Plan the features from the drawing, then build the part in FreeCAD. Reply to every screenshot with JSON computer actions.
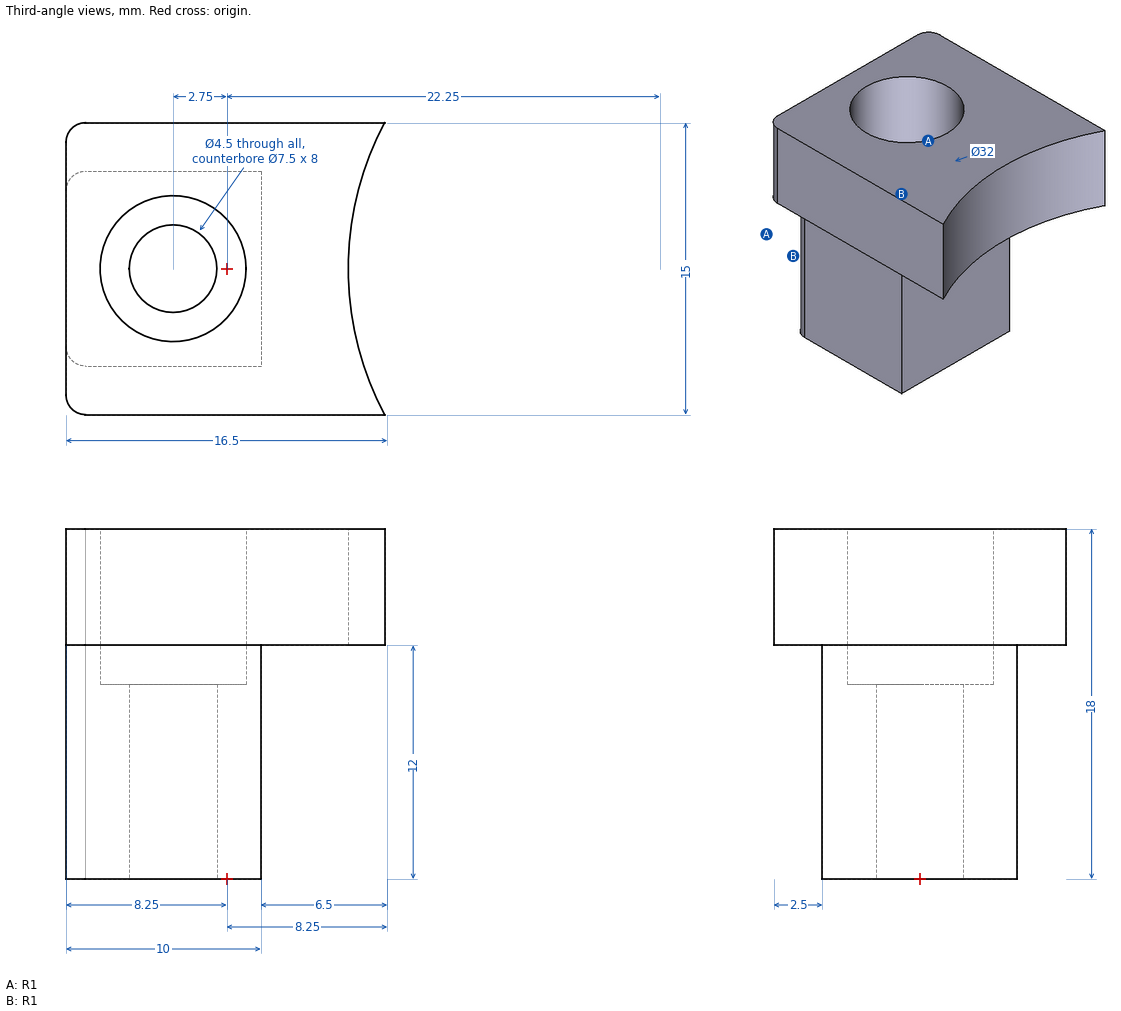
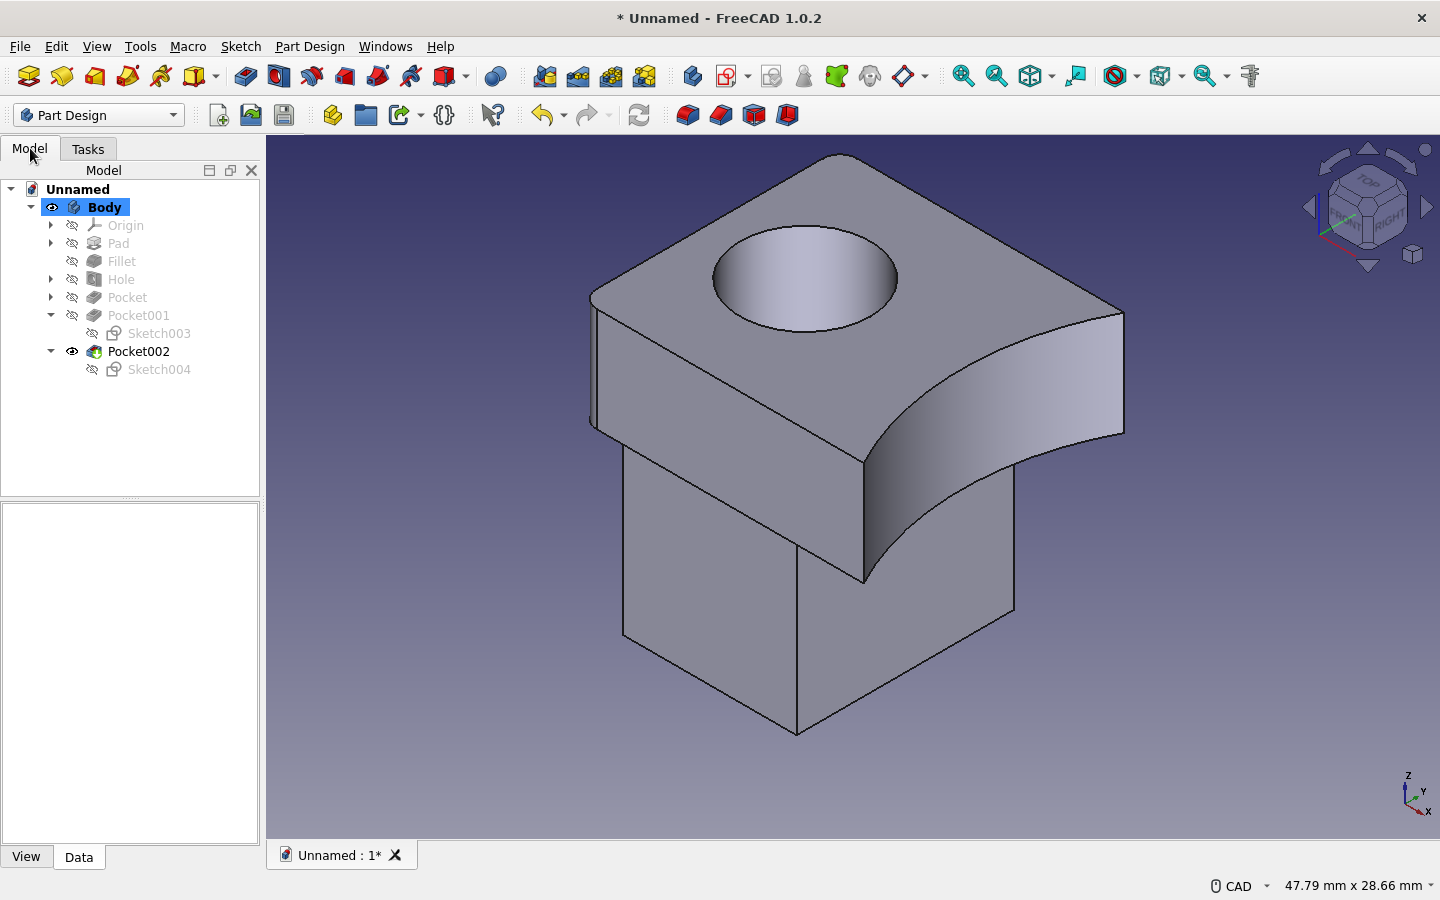
{"action": "left_click", "coordinate": [117, 351]}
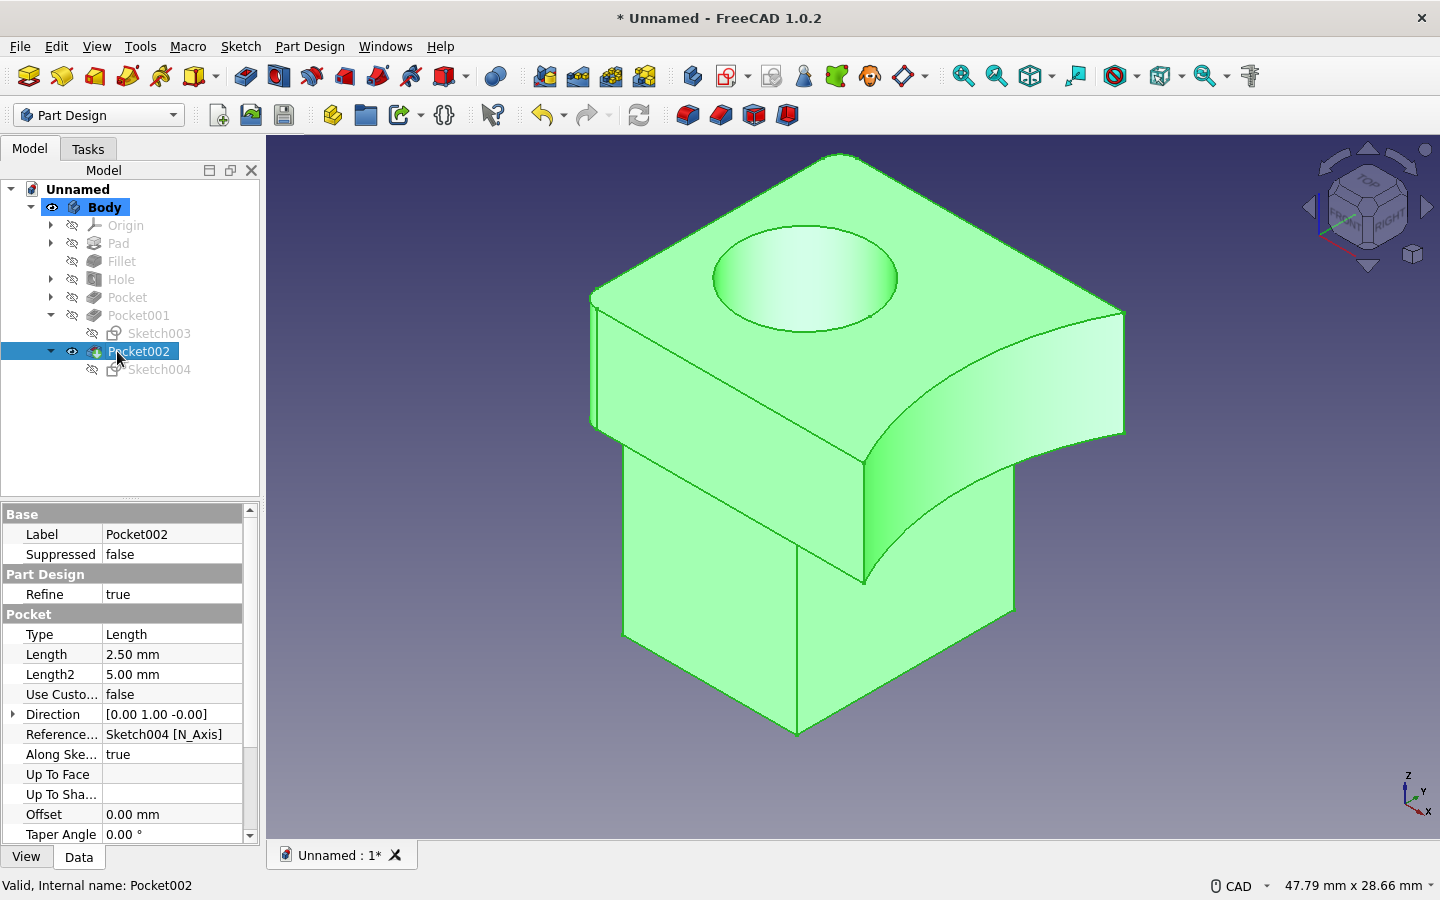
{"action": "left_click", "coordinate": [545, 76]}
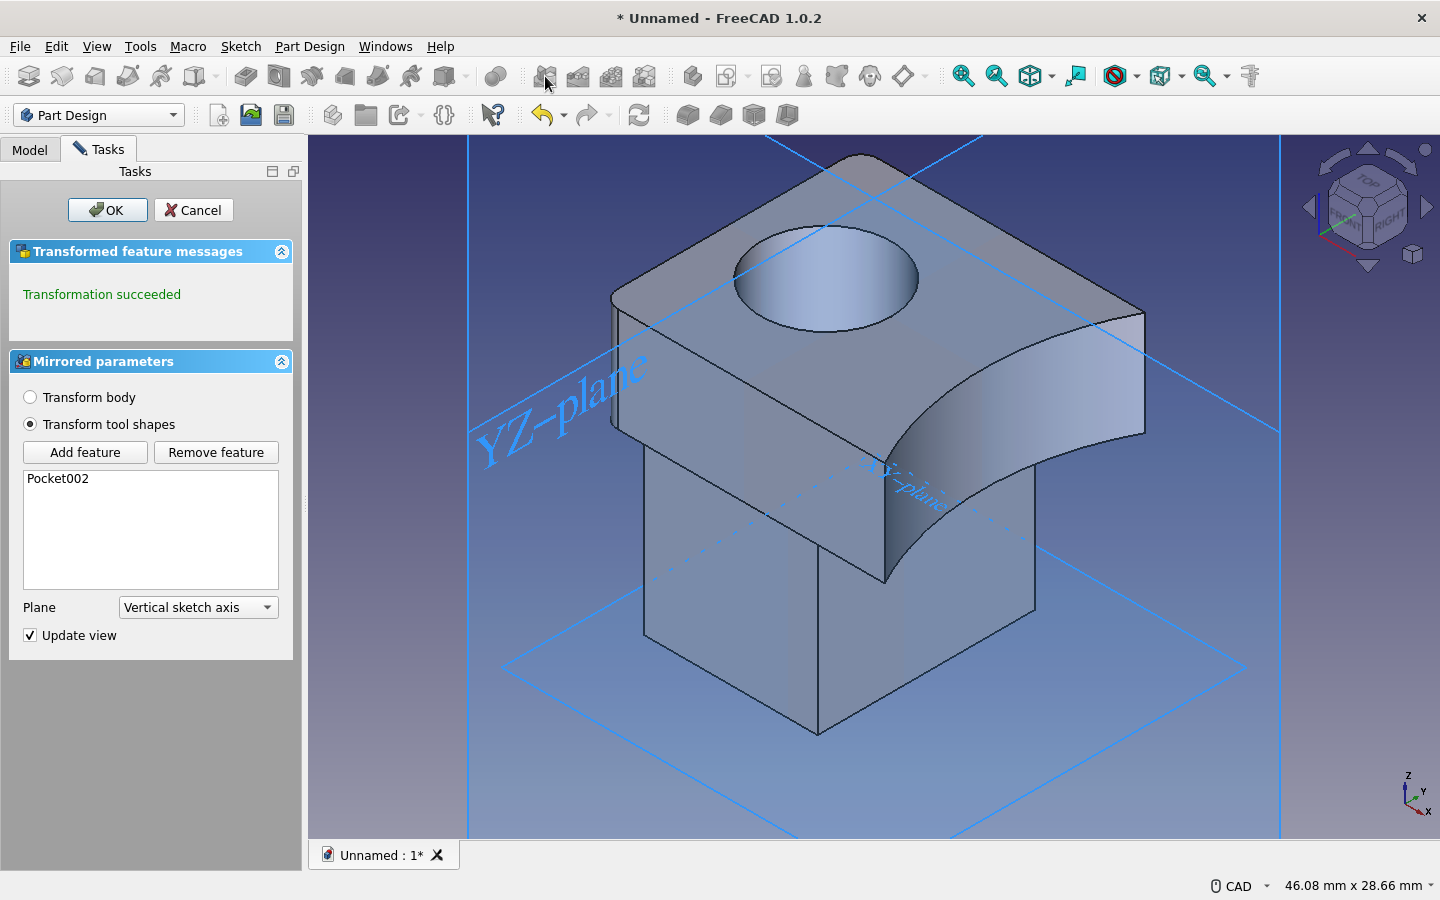
{"action": "left_click", "coordinate": [199, 608]}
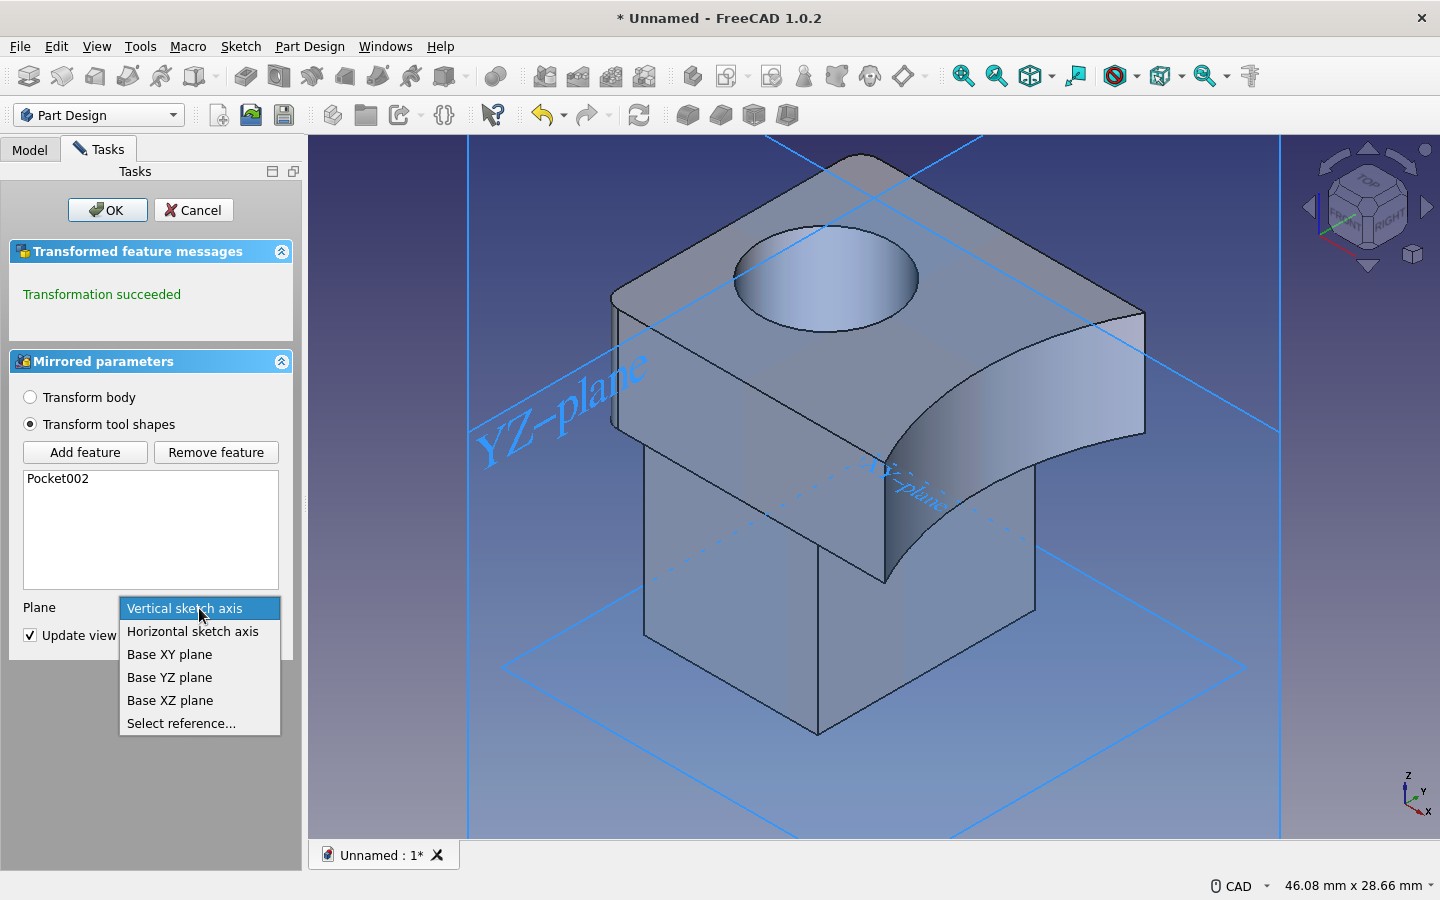
{"action": "left_click", "coordinate": [198, 700]}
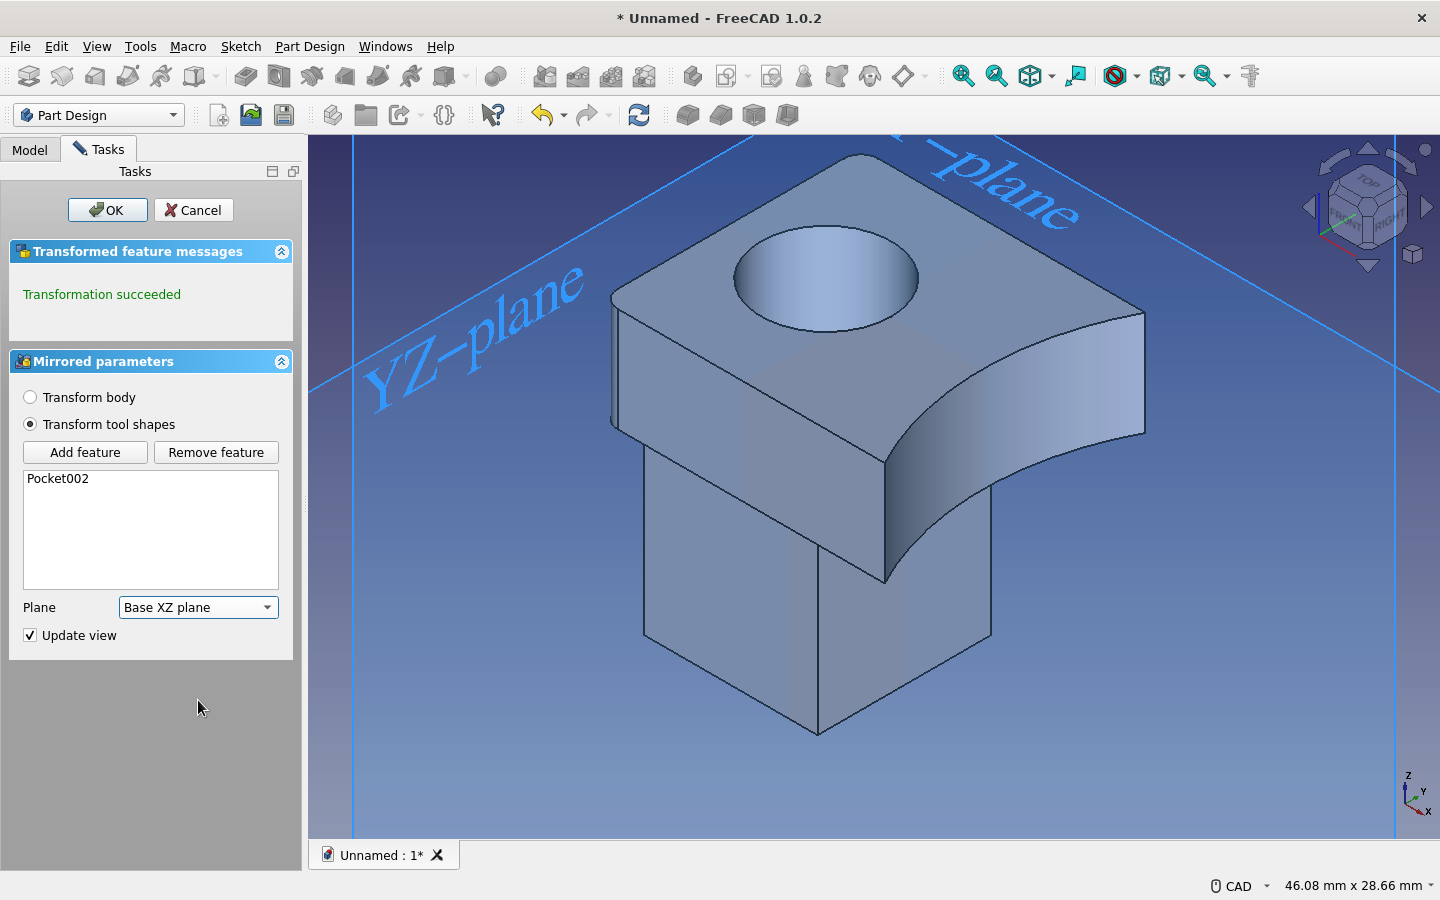
{"action": "left_click", "coordinate": [108, 210]}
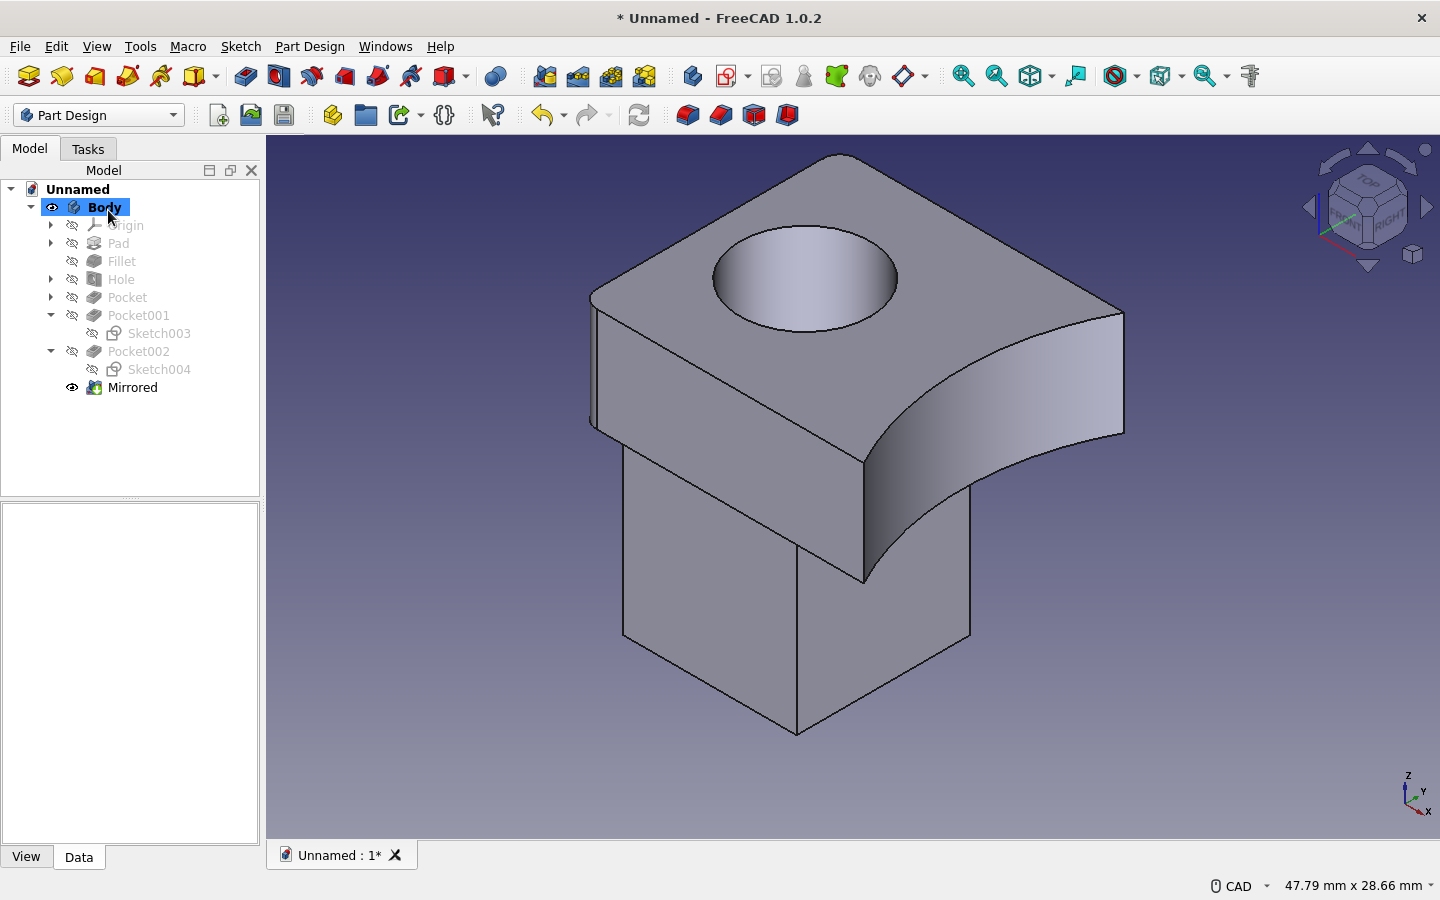
{"action": "key", "text": "2"}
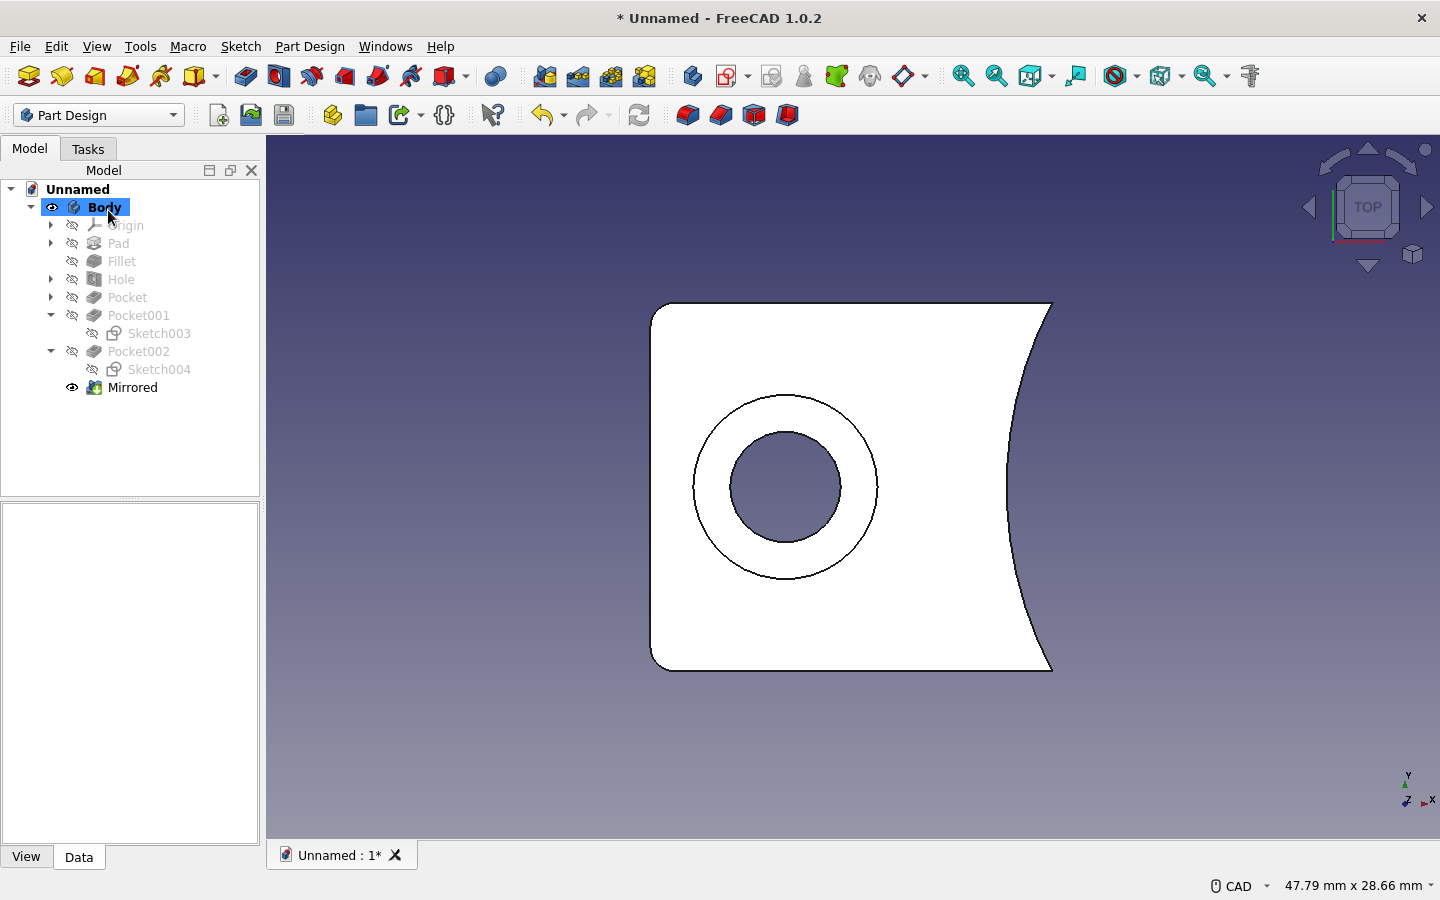
{"action": "key", "text": "0"}